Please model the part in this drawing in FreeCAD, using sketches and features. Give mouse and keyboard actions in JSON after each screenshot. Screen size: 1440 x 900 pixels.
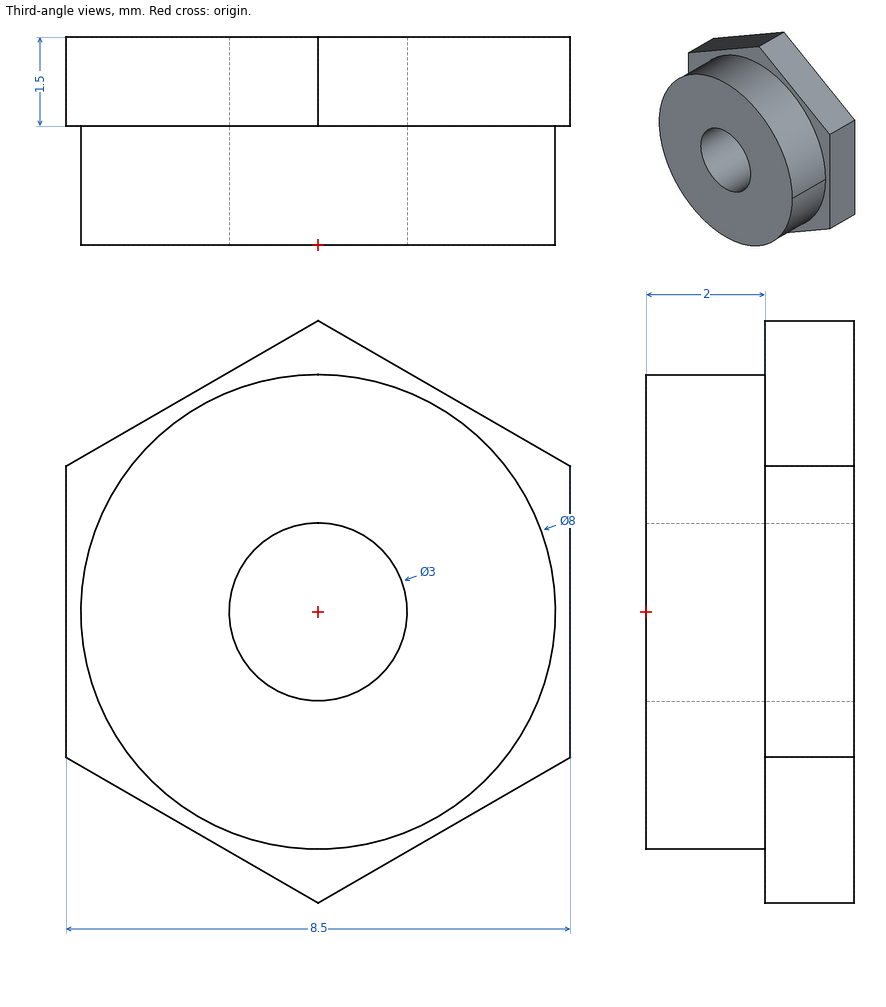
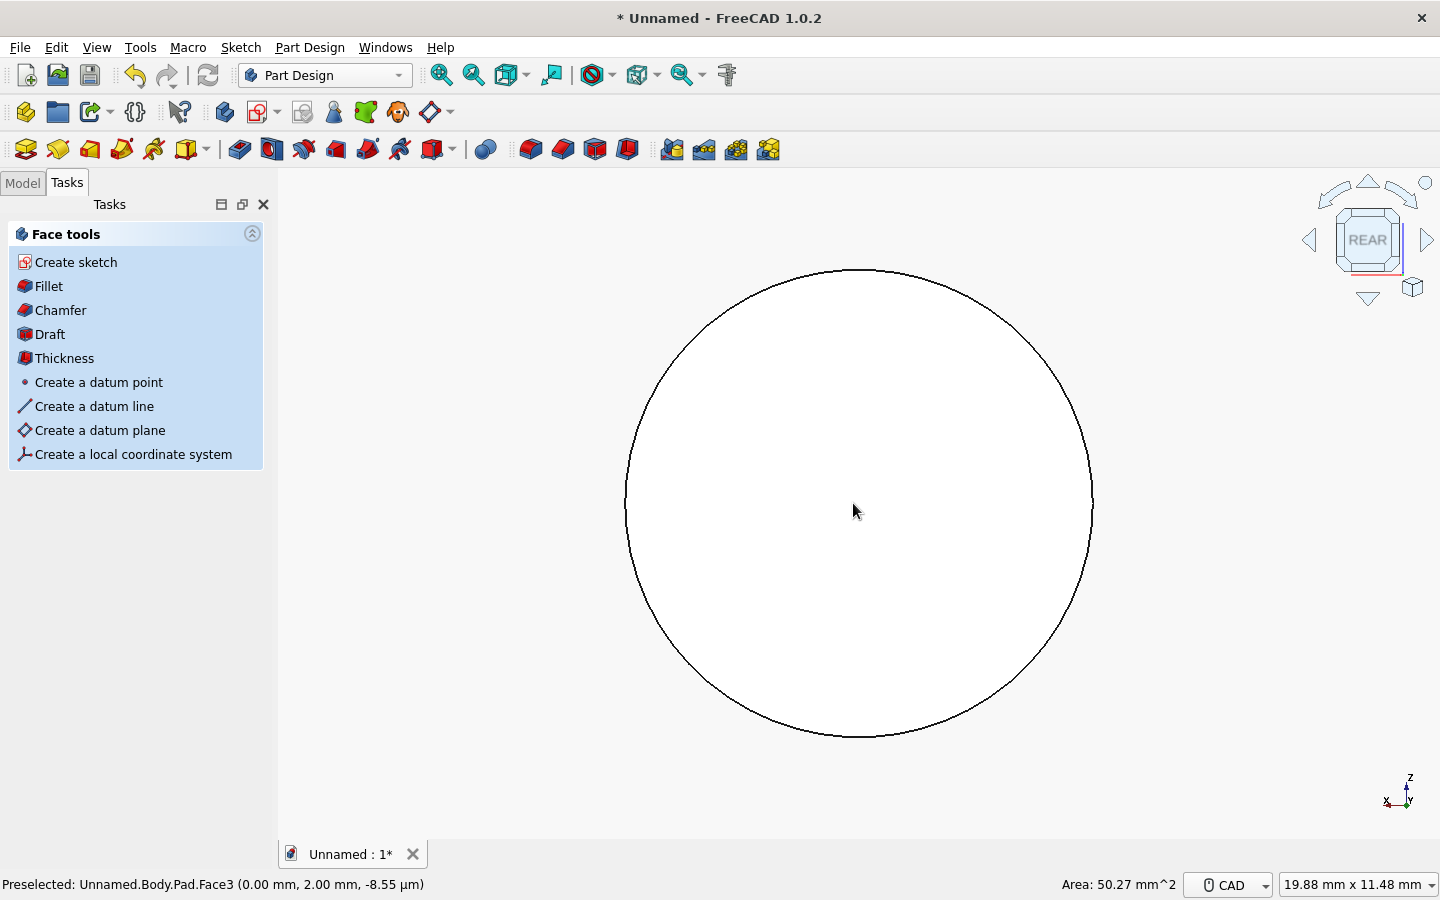
{"action": "left_click", "coordinate": [258, 112]}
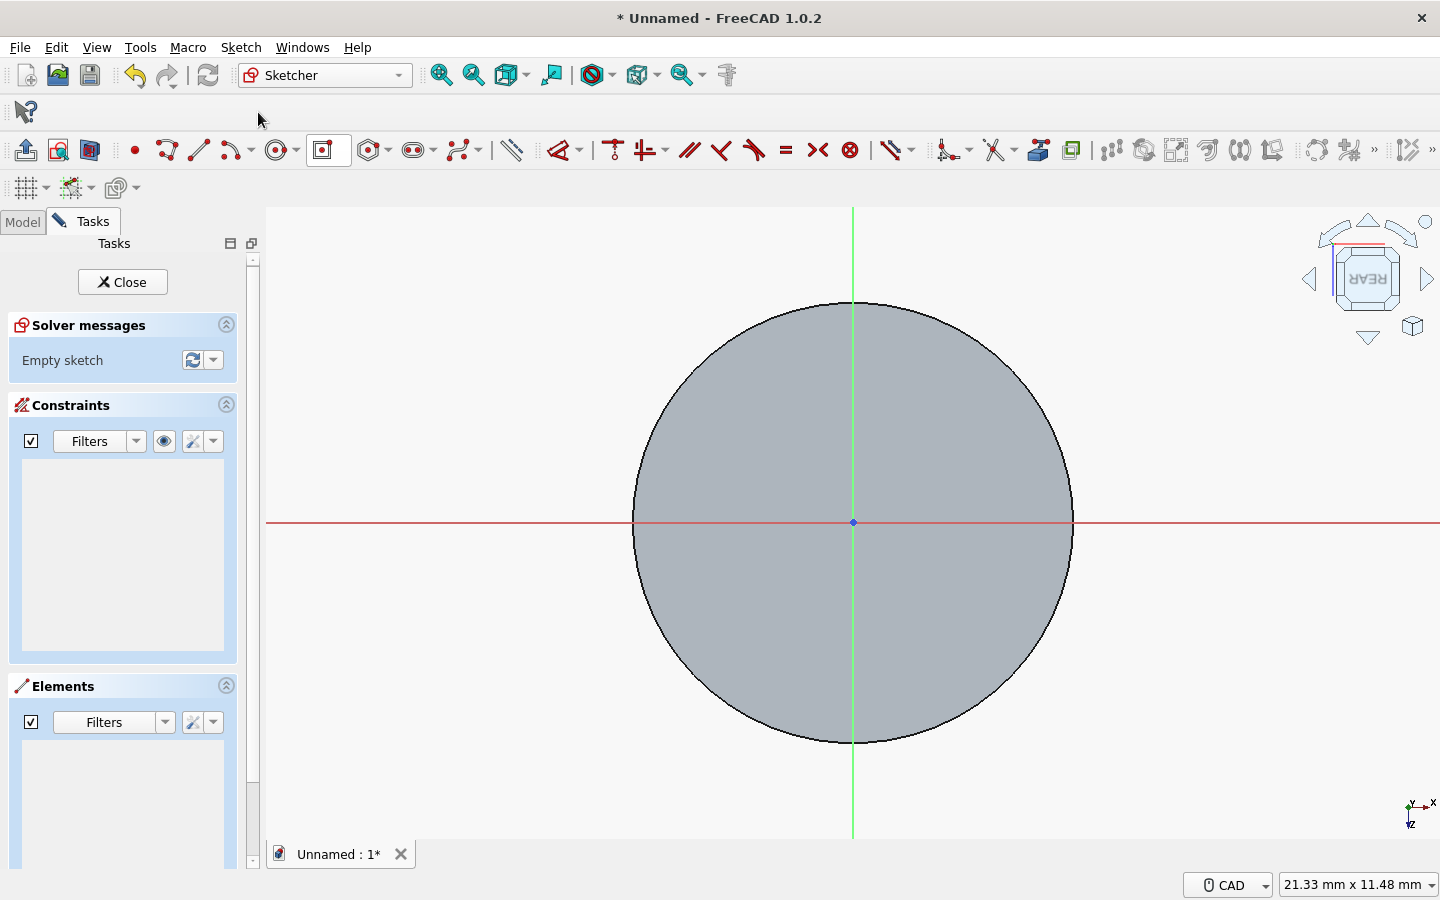
{"action": "scroll", "coordinate": [475, 523], "scroll_direction": "down", "scroll_amount": 1}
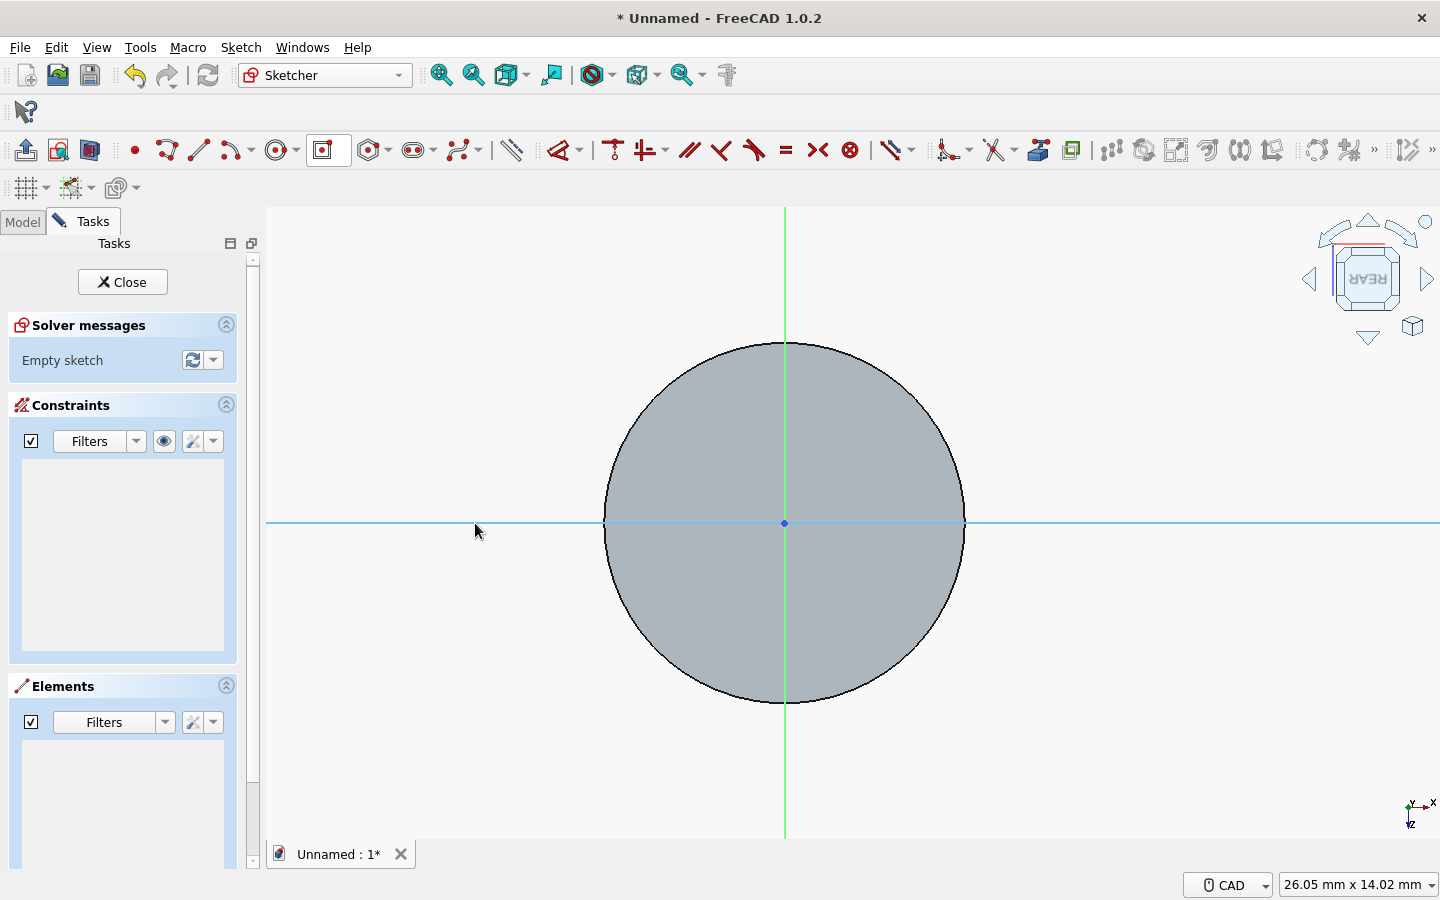
{"action": "key", "text": "g p 6"}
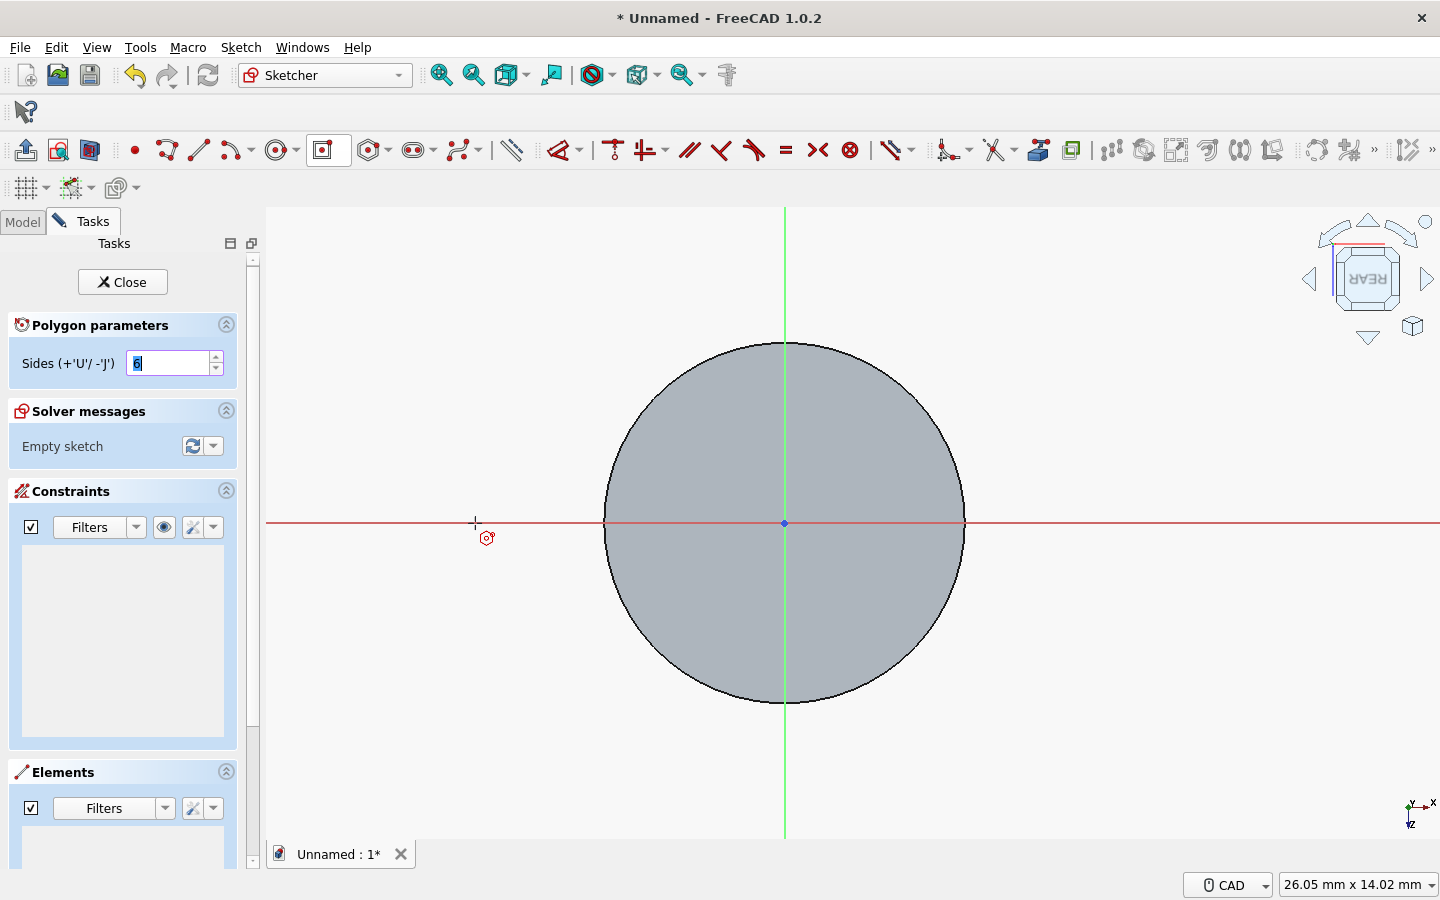
{"action": "left_click", "coordinate": [785, 523]}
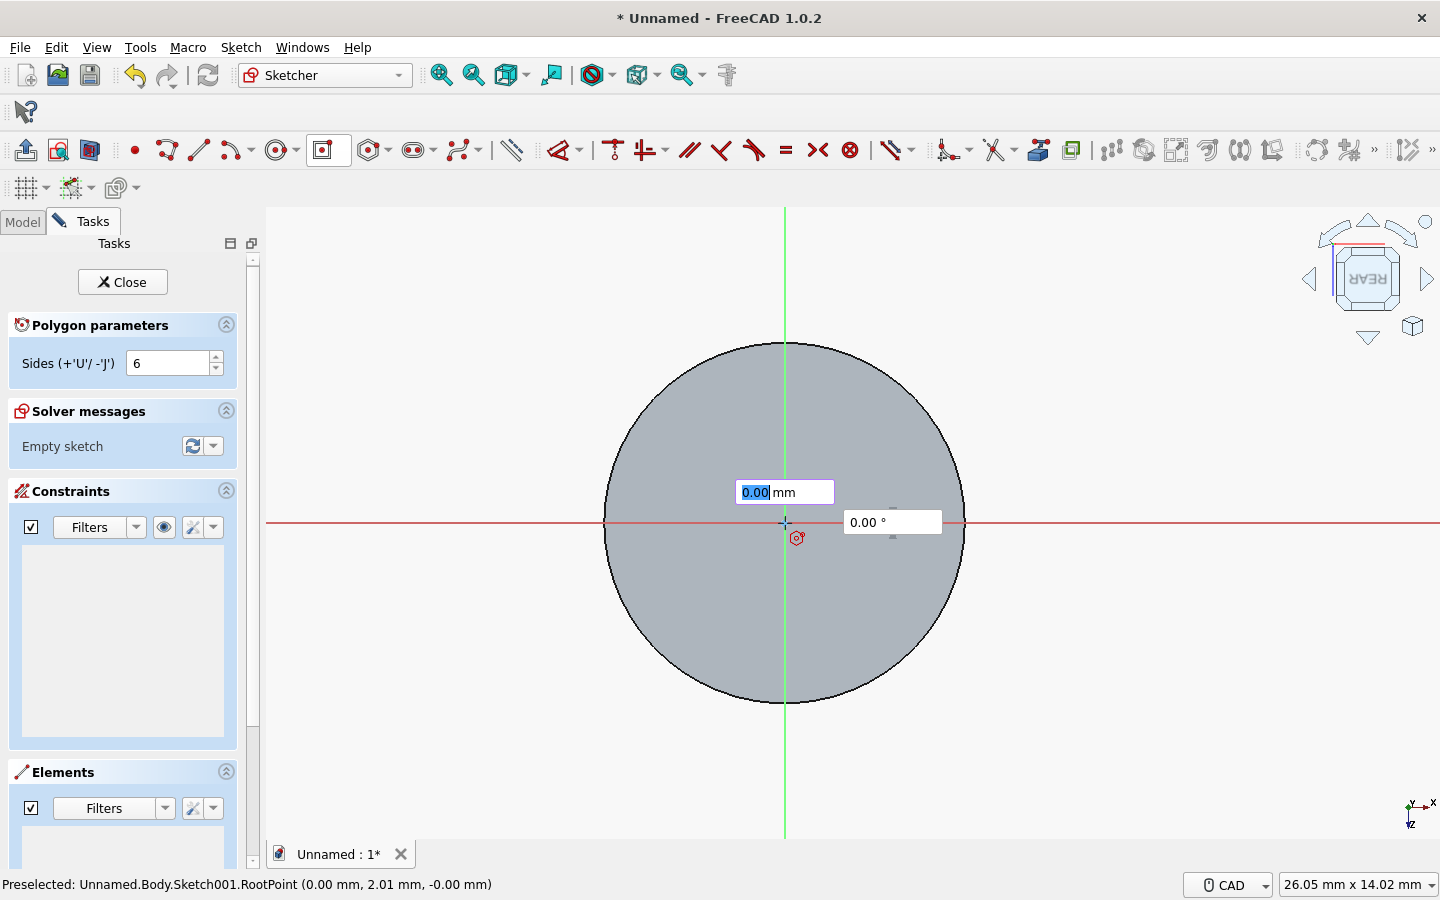
{"action": "left_click", "coordinate": [785, 302]}
{"action": "right_click", "coordinate": [785, 302]}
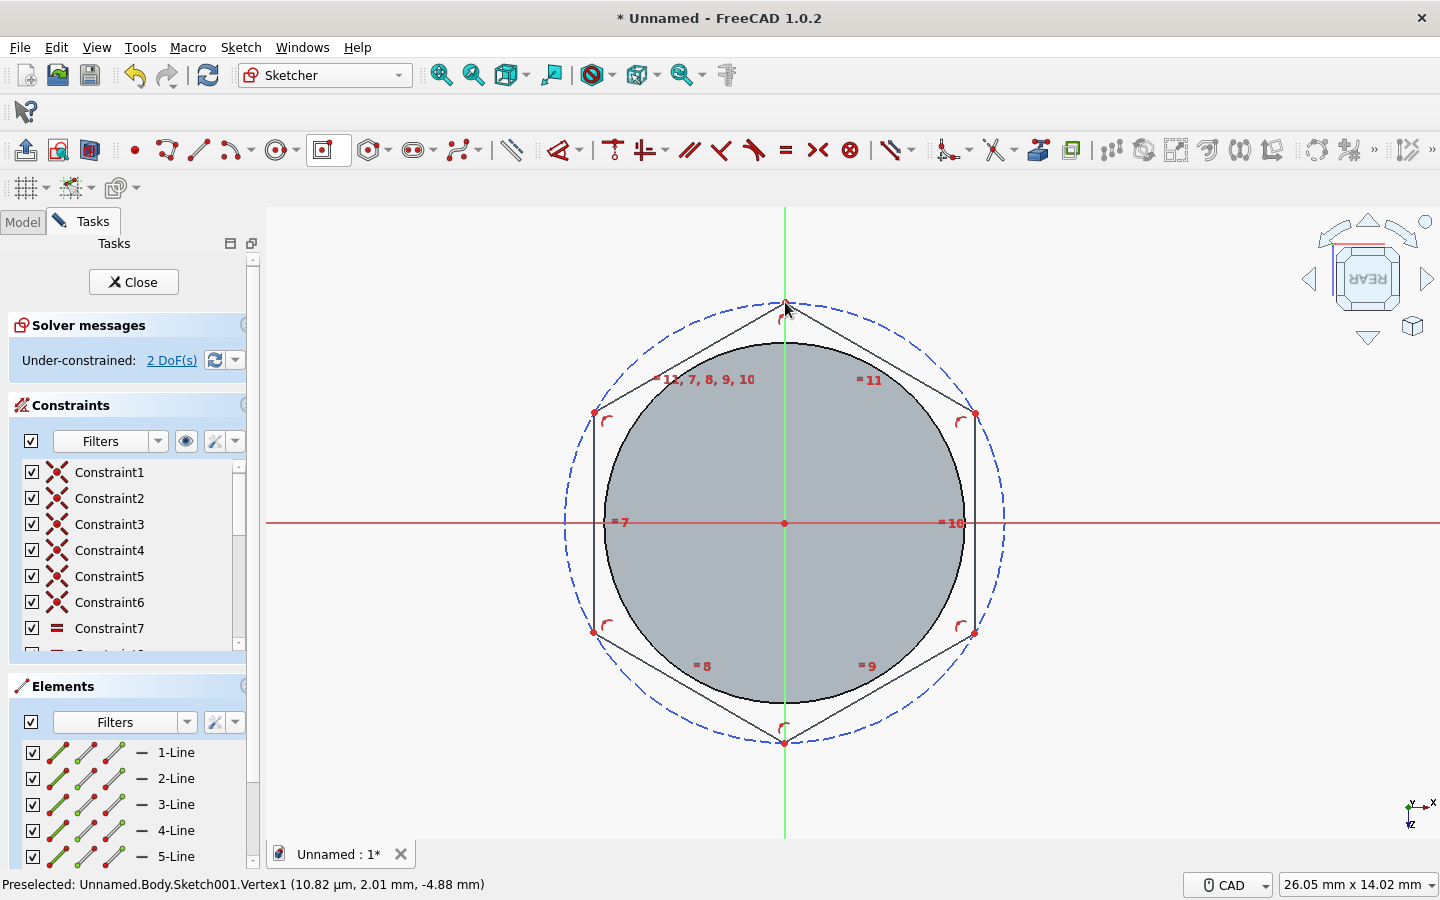
{"action": "left_click", "coordinate": [594, 479]}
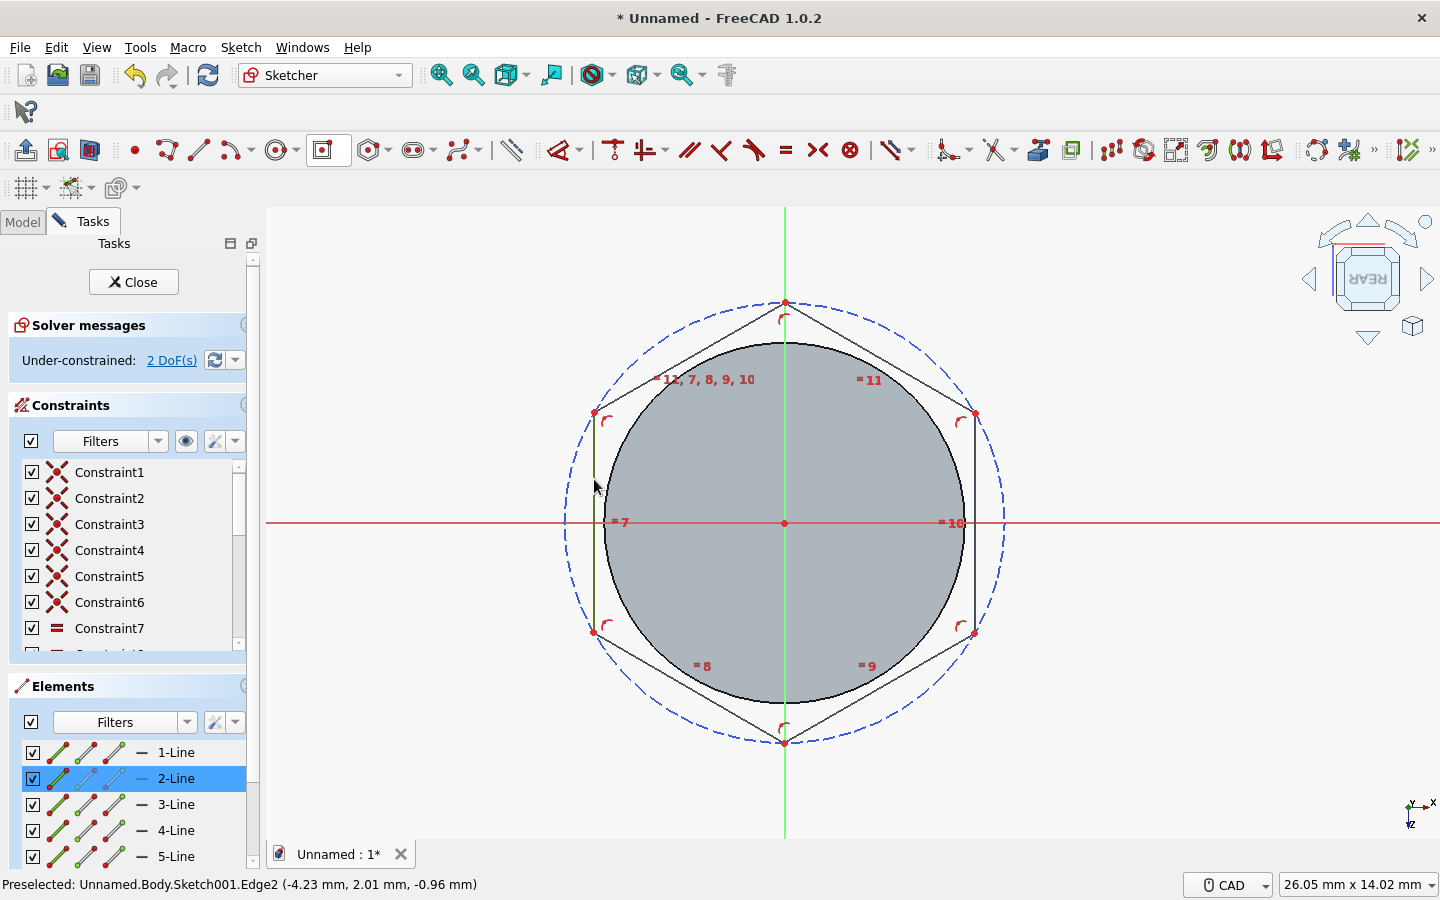
{"action": "key", "text": "v"}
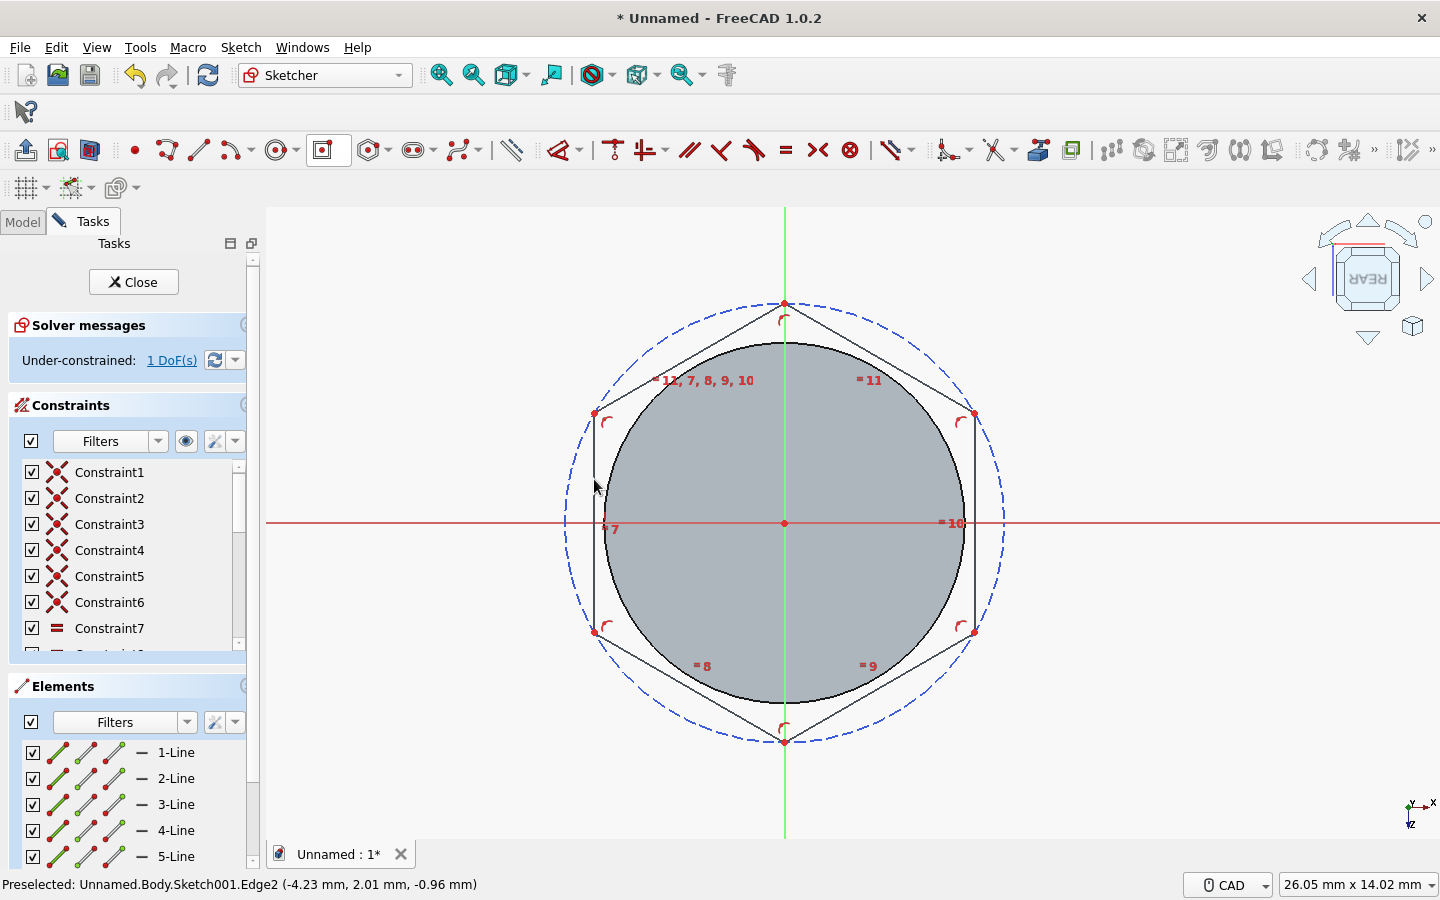
{"action": "key", "text": "d"}